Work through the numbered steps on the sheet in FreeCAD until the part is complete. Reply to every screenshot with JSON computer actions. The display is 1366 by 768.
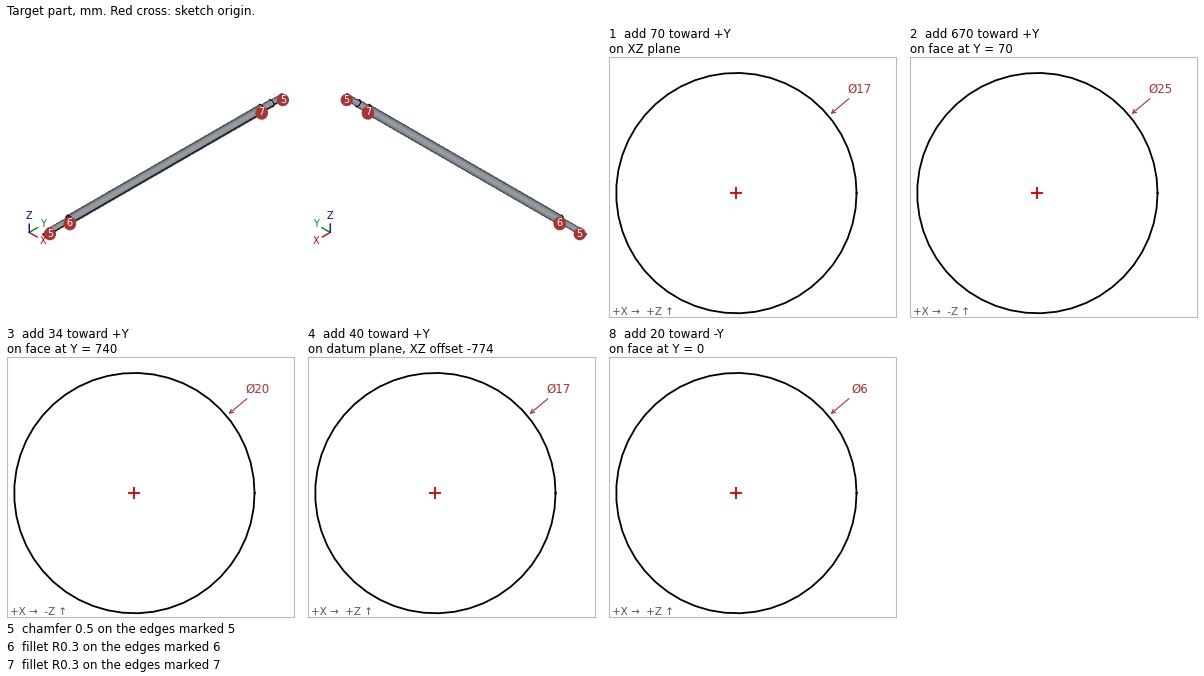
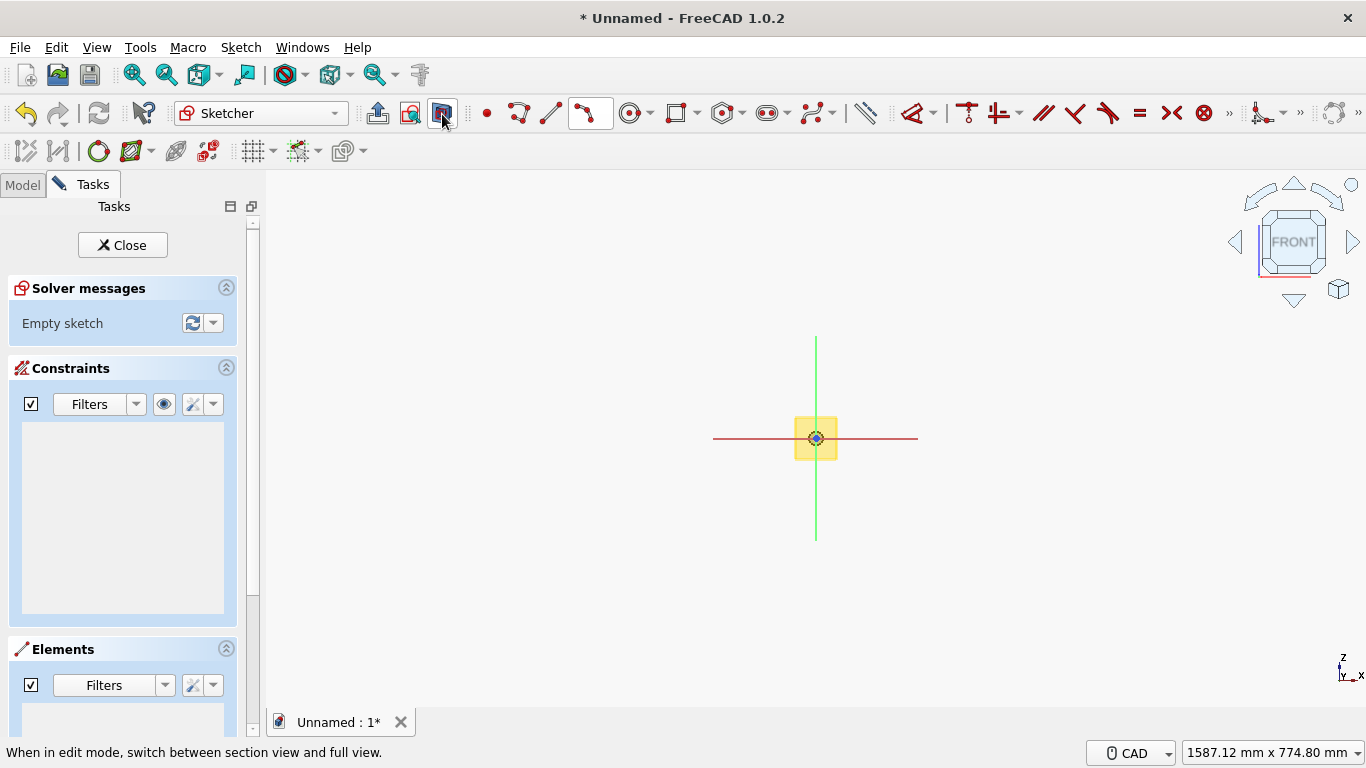
{"action": "scroll", "coordinate": [820, 439], "scroll_direction": "up", "scroll_amount": 15}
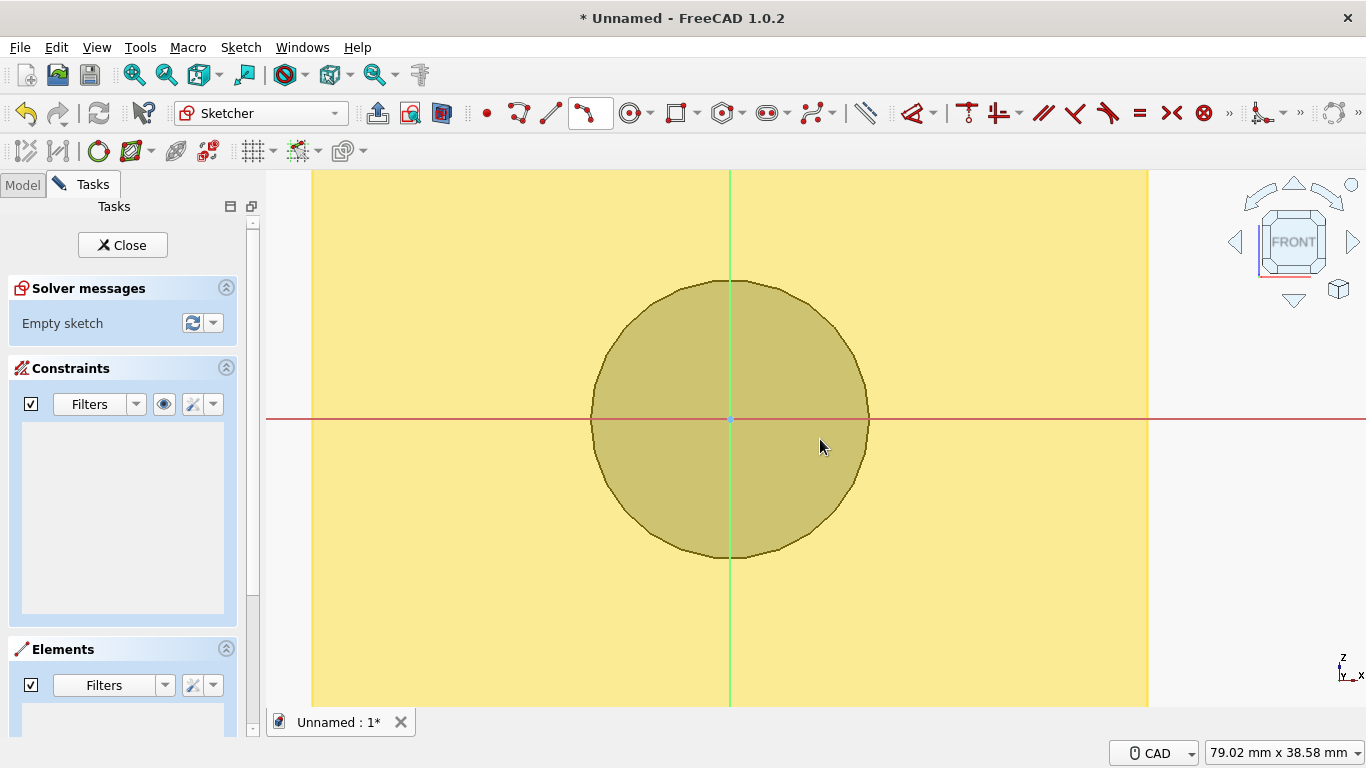
{"action": "scroll", "coordinate": [695, 381], "scroll_direction": "up", "scroll_amount": 2}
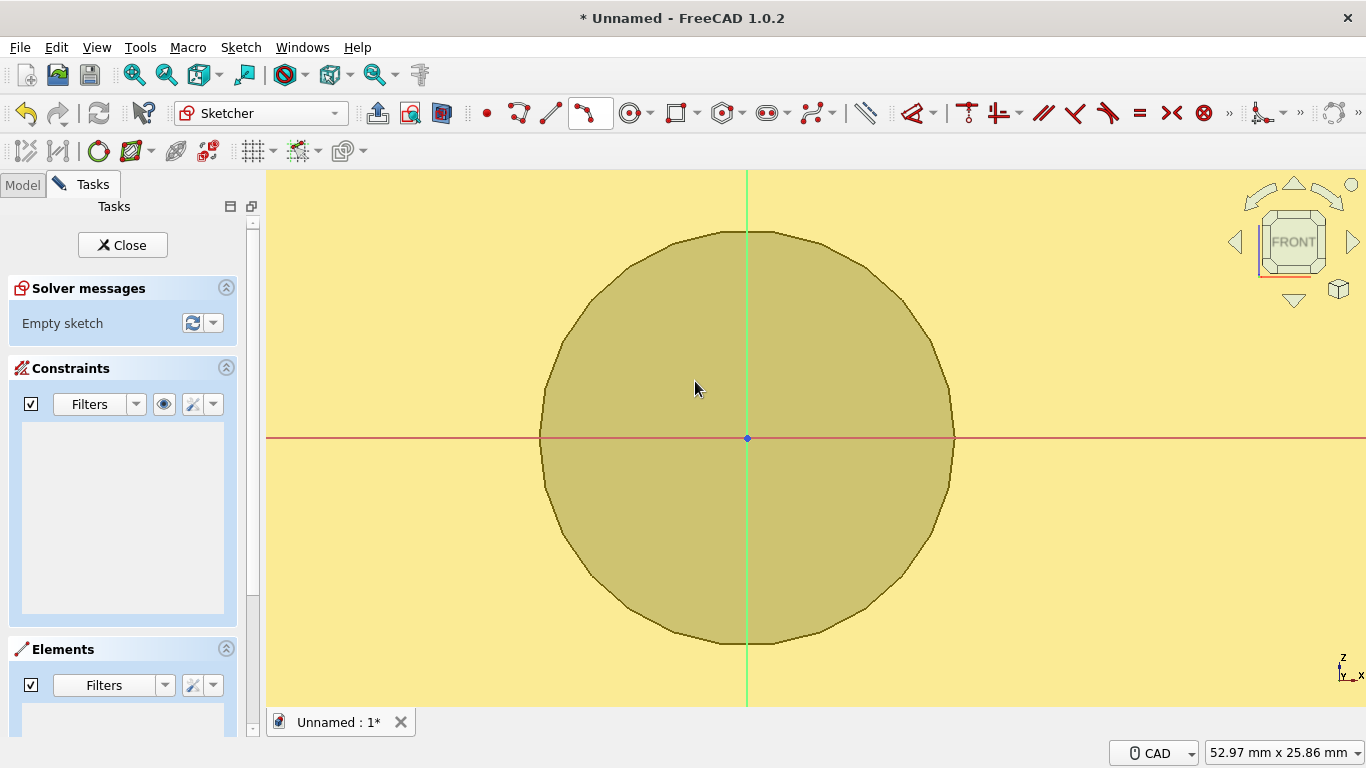
{"action": "key", "text": "g c"}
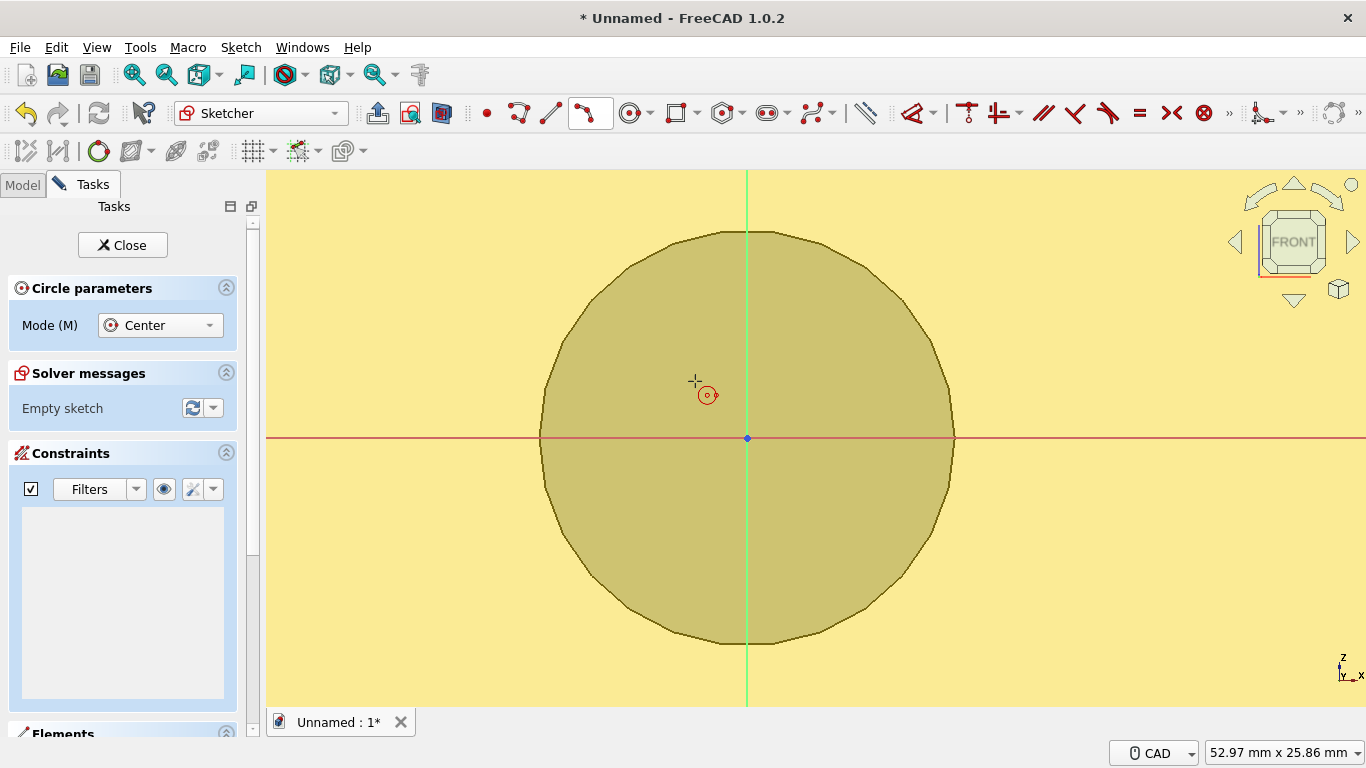
{"action": "left_click", "coordinate": [747, 438]}
{"action": "left_click", "coordinate": [872, 313]}
{"action": "key", "text": "Escape"}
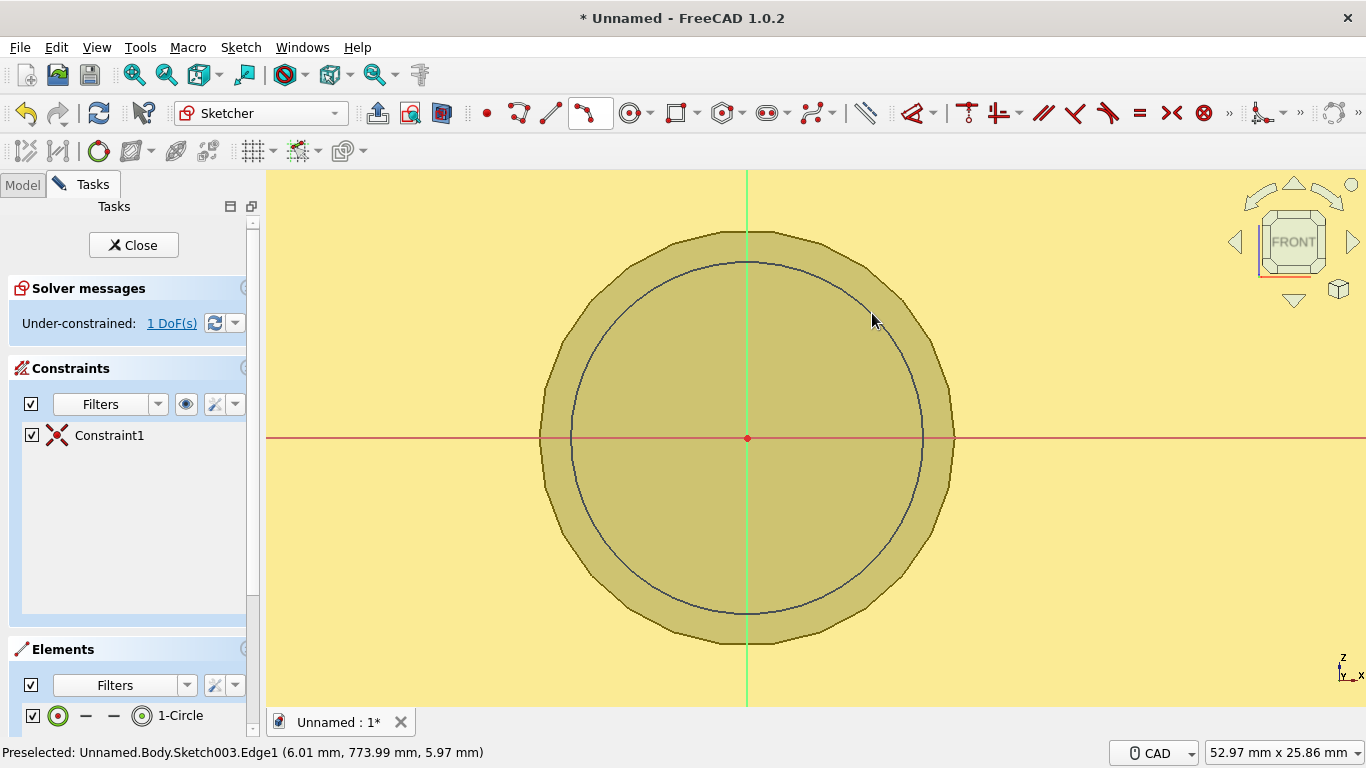
{"action": "left_click", "coordinate": [912, 114]}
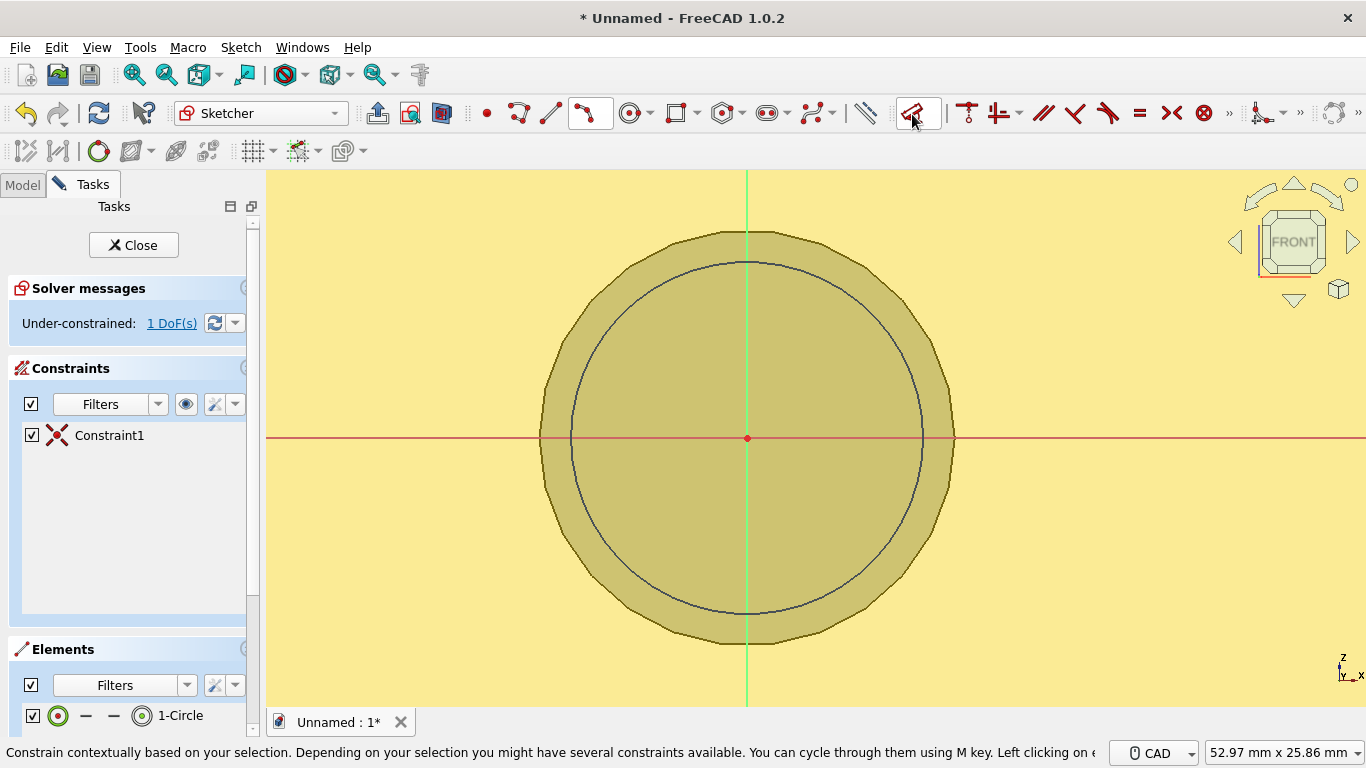
{"action": "left_click", "coordinate": [871, 313]}
{"action": "left_click", "coordinate": [894, 290]}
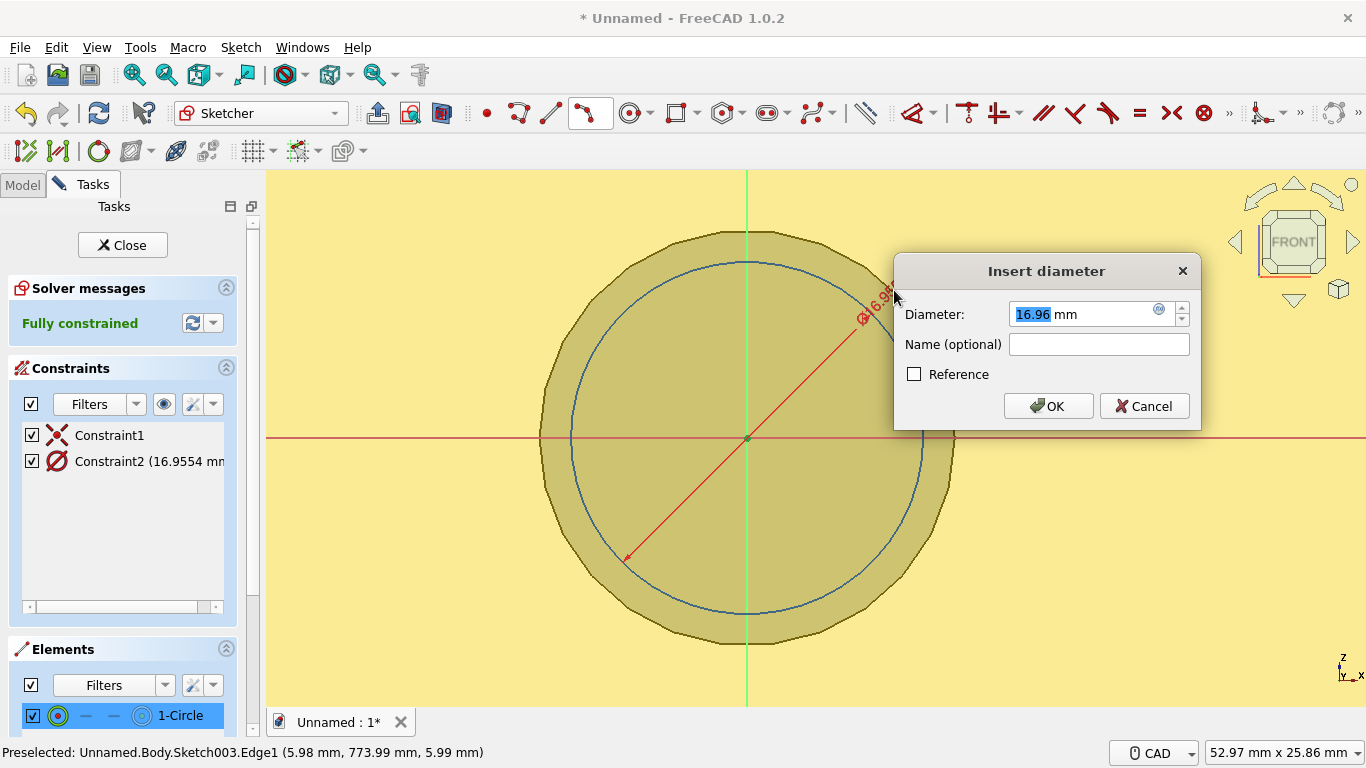
{"action": "type", "text": "17"}
{"action": "key", "text": "Return"}
{"action": "key", "text": "Escape"}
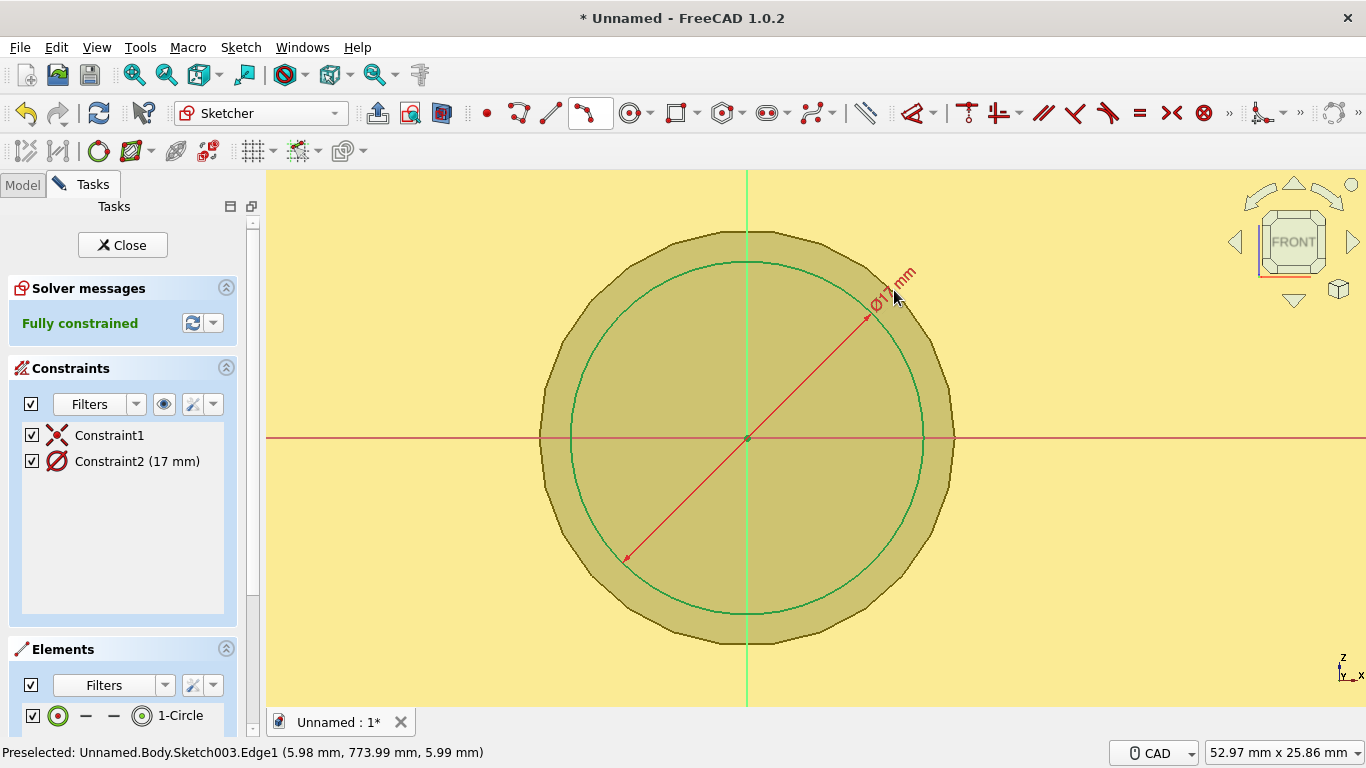
{"action": "left_click", "coordinate": [123, 245]}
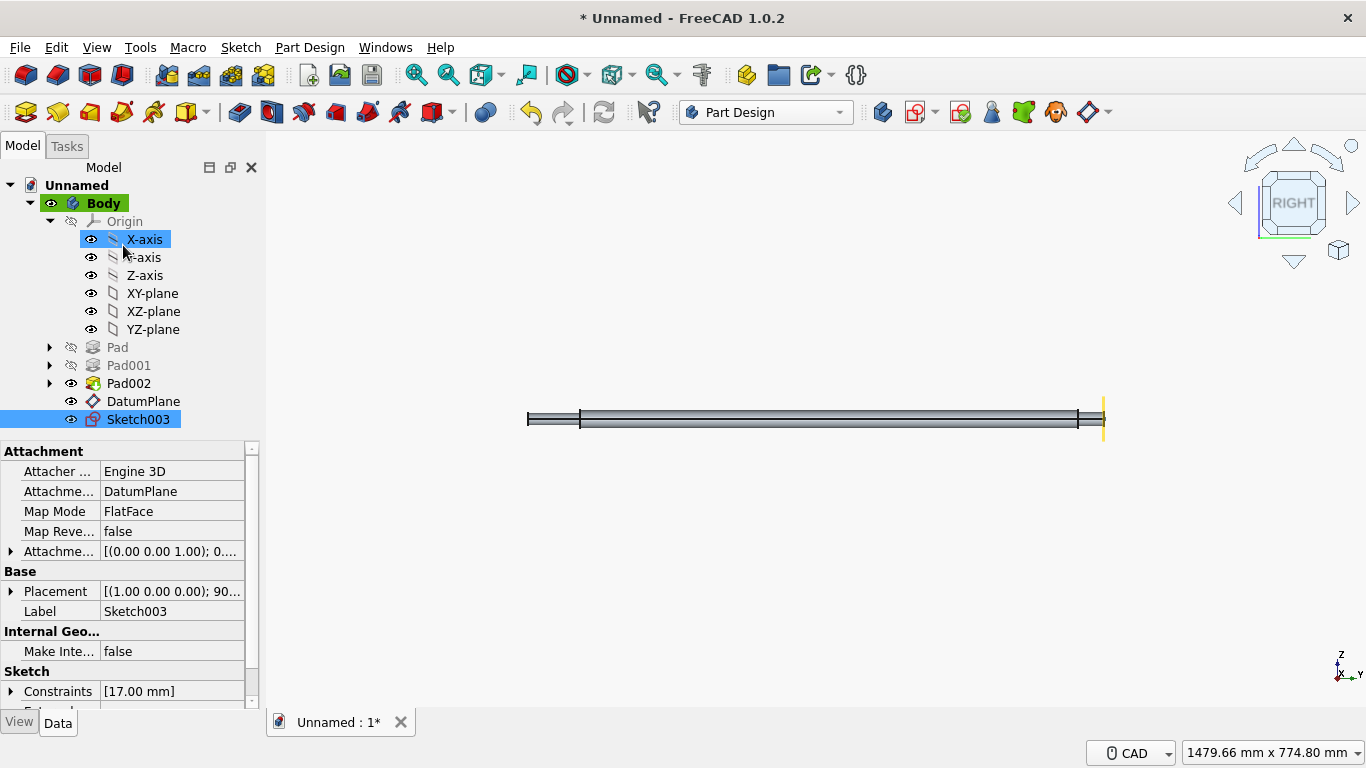
{"action": "left_click", "coordinate": [26, 112]}